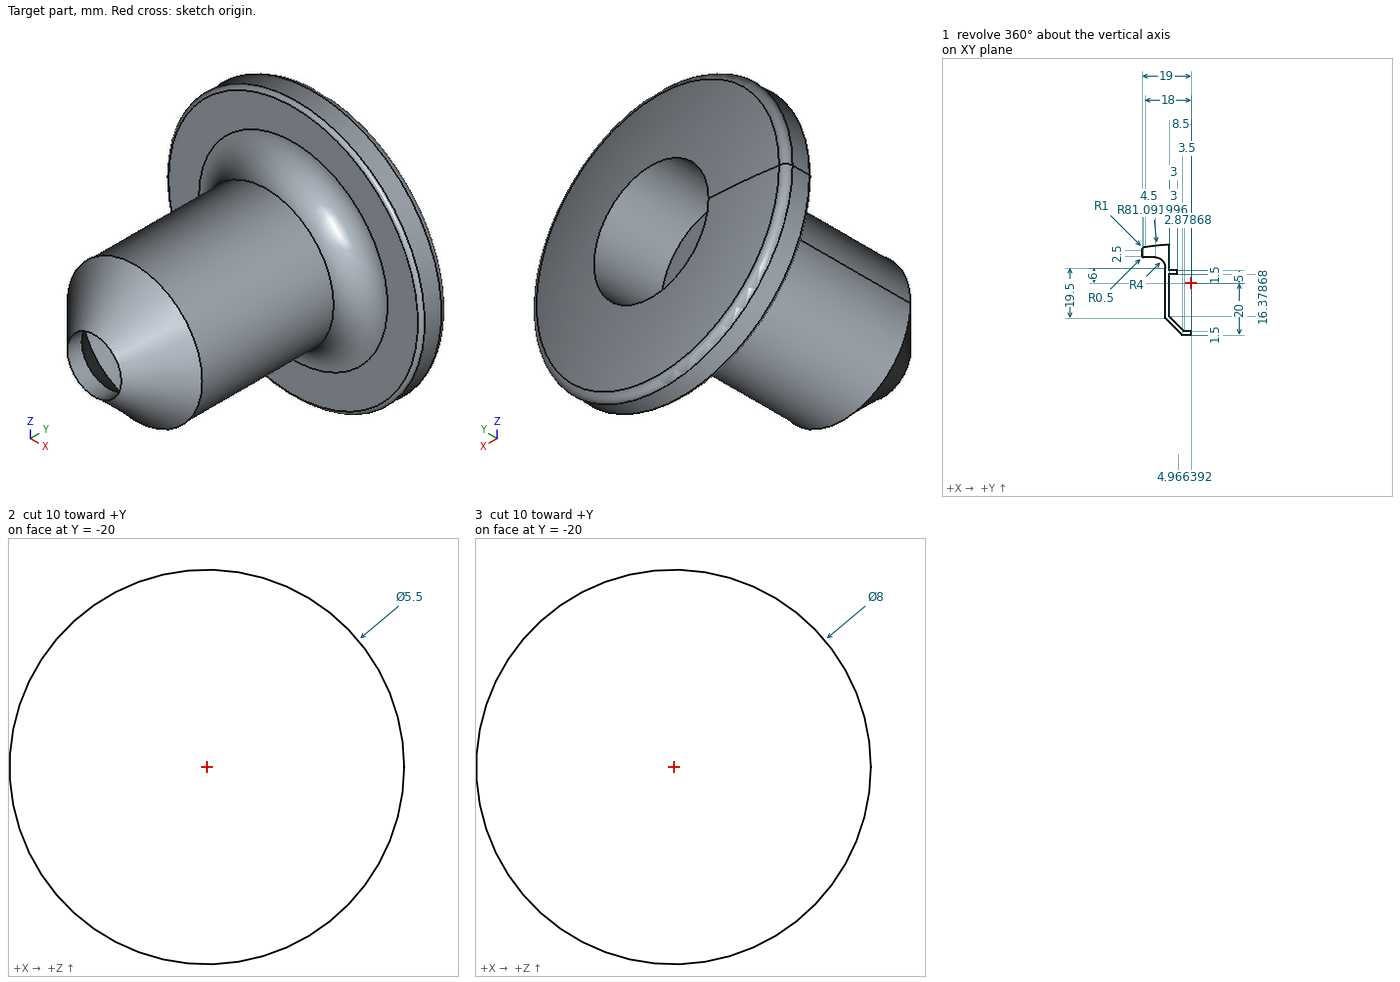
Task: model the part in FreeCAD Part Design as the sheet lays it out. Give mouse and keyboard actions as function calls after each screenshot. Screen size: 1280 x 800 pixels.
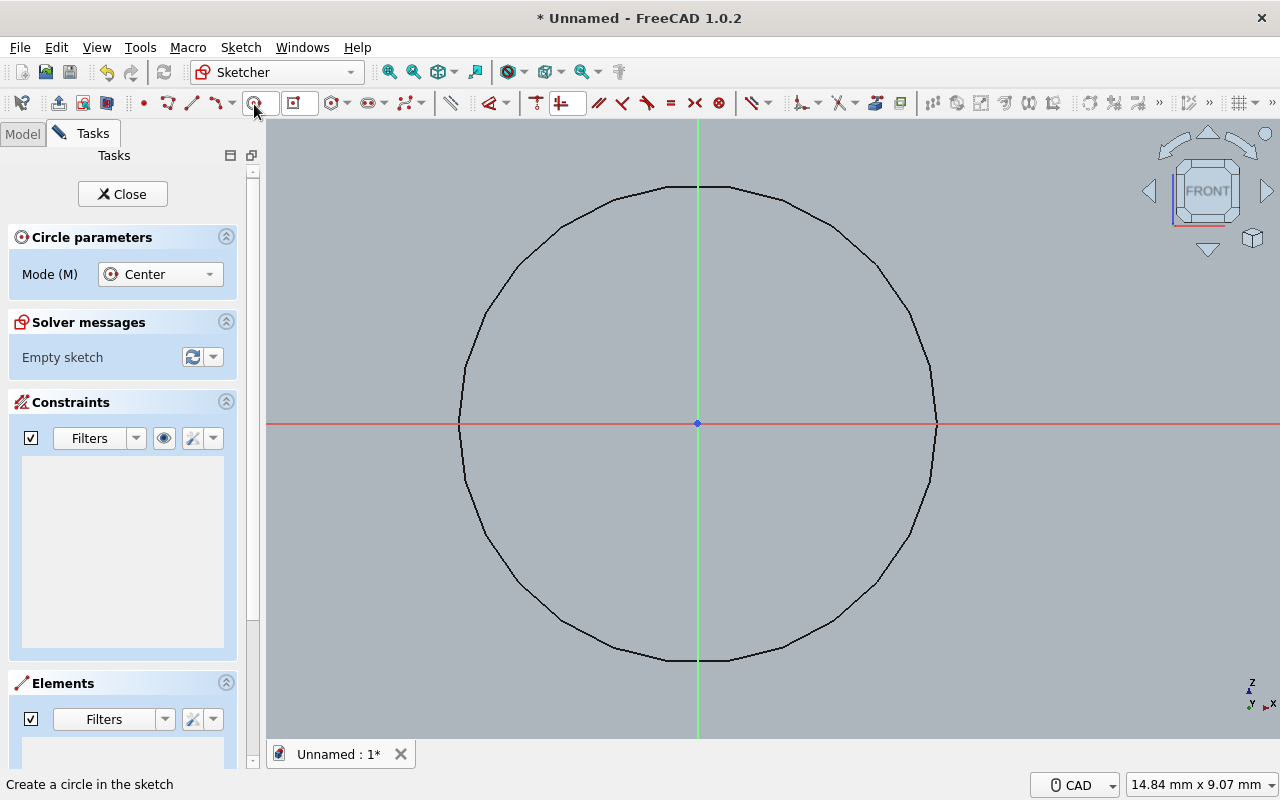
click(698, 424)
move(831, 291)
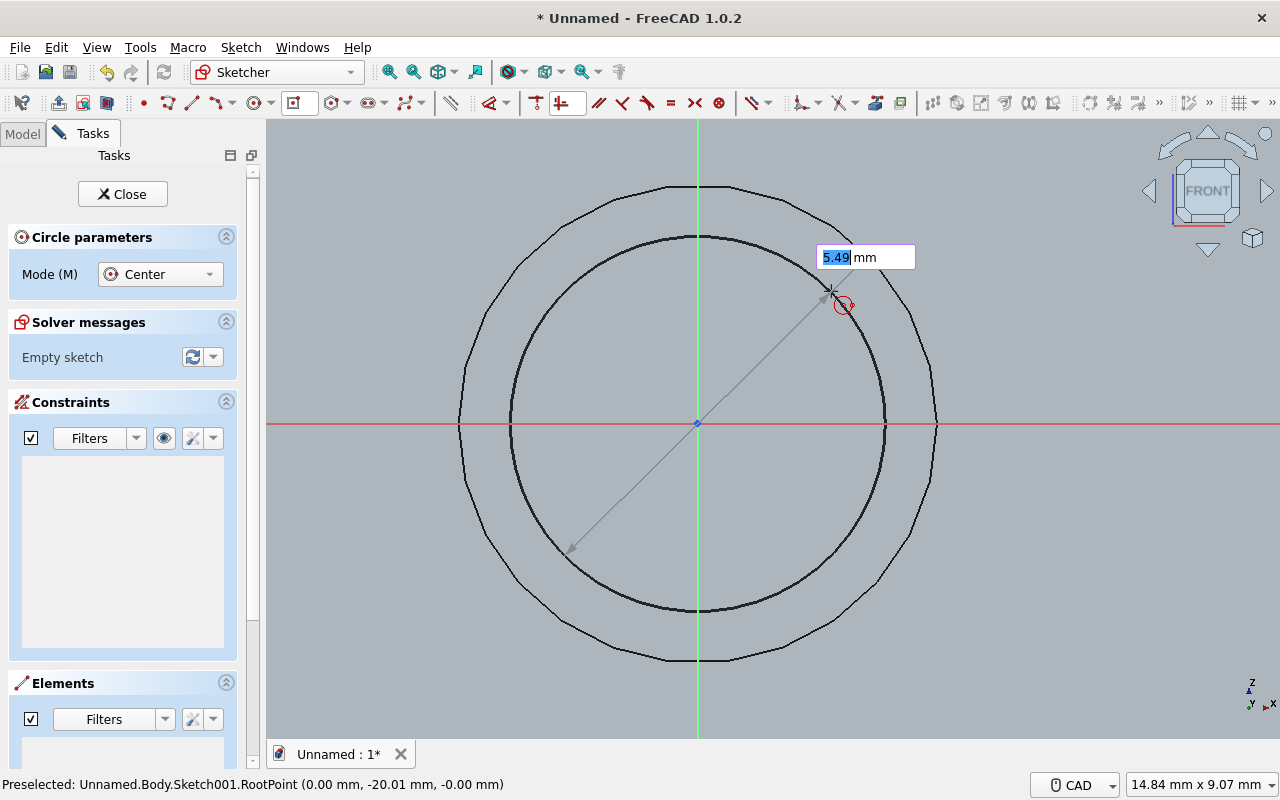
text(5.5)
key(Return)
key(Escape)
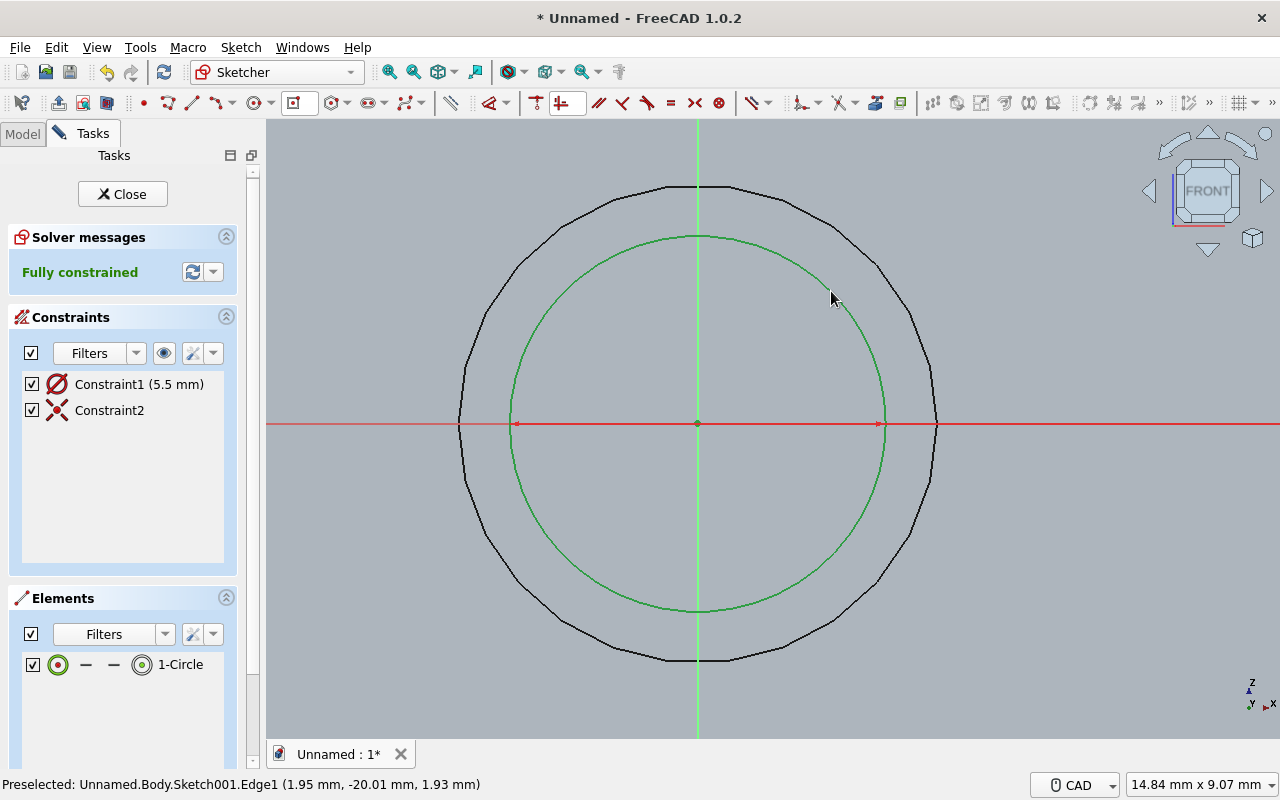
click(123, 194)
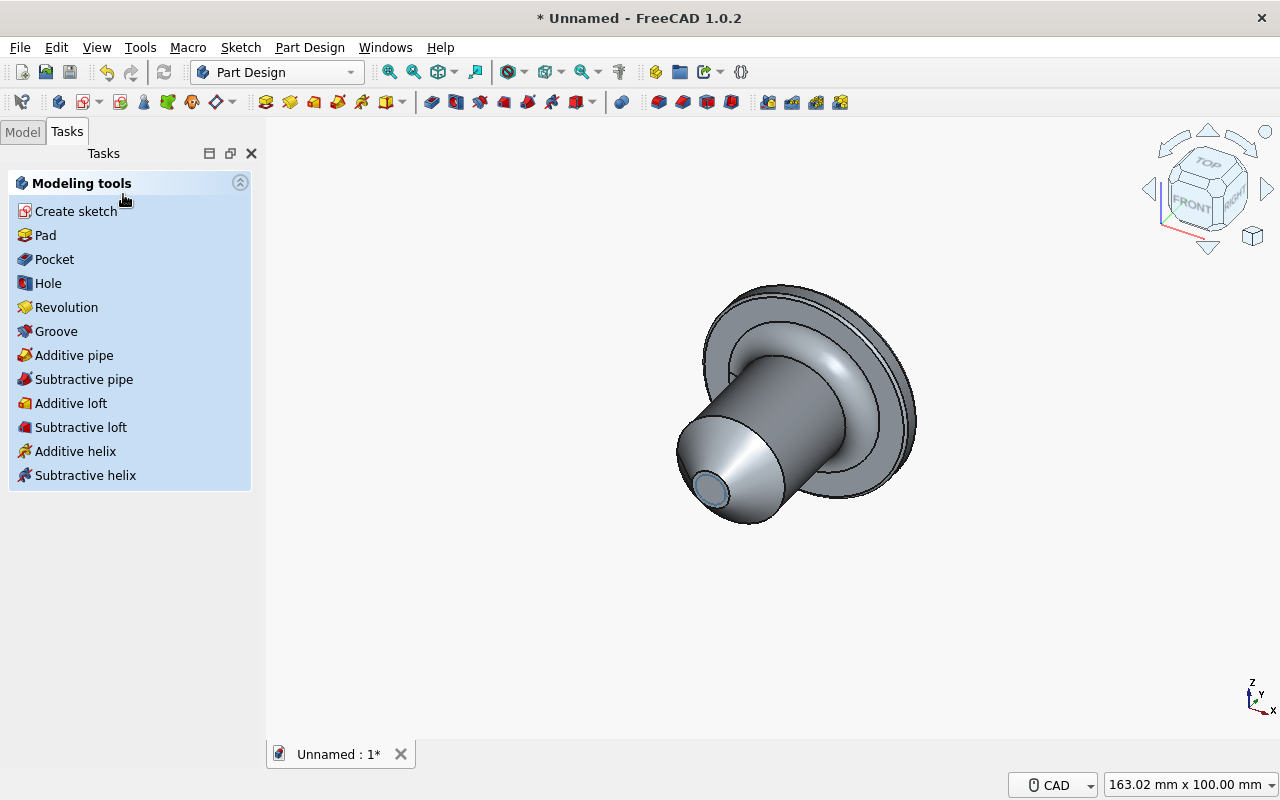
click(432, 102)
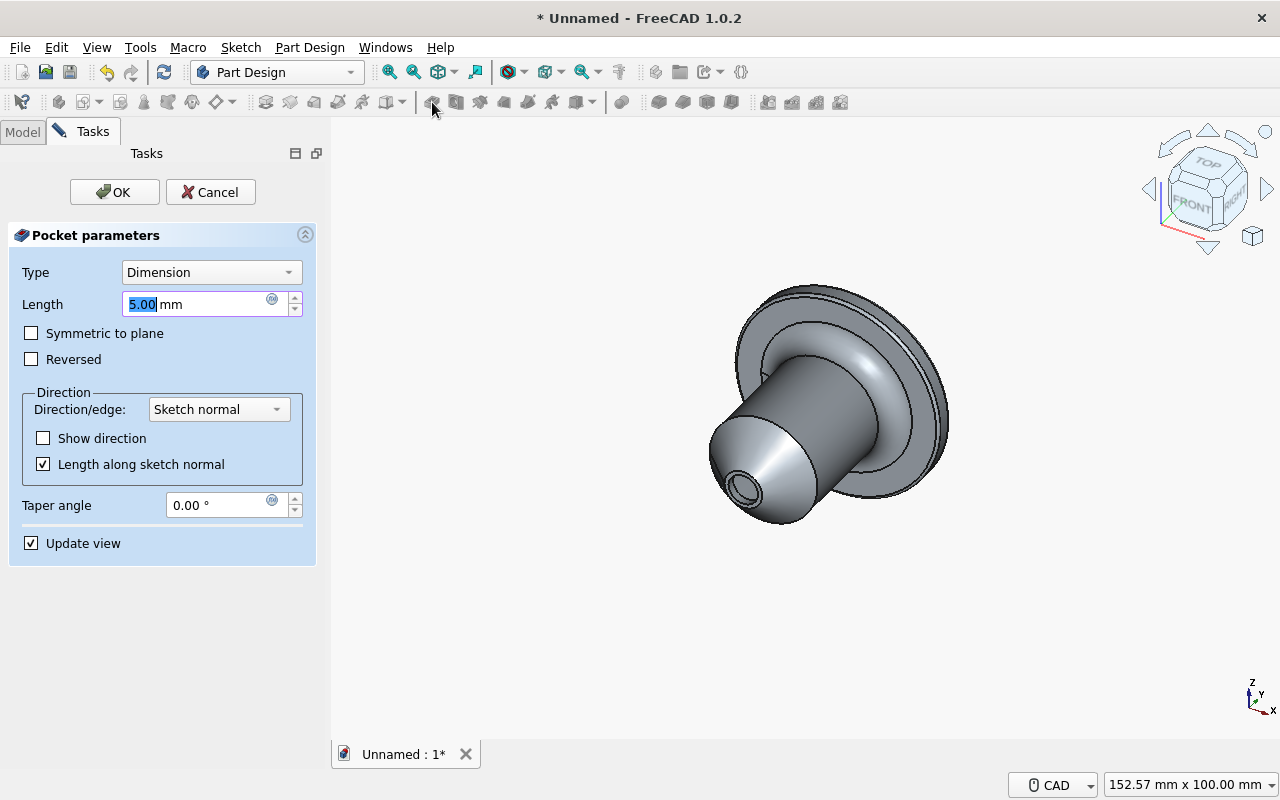
text(10)
key(Tab)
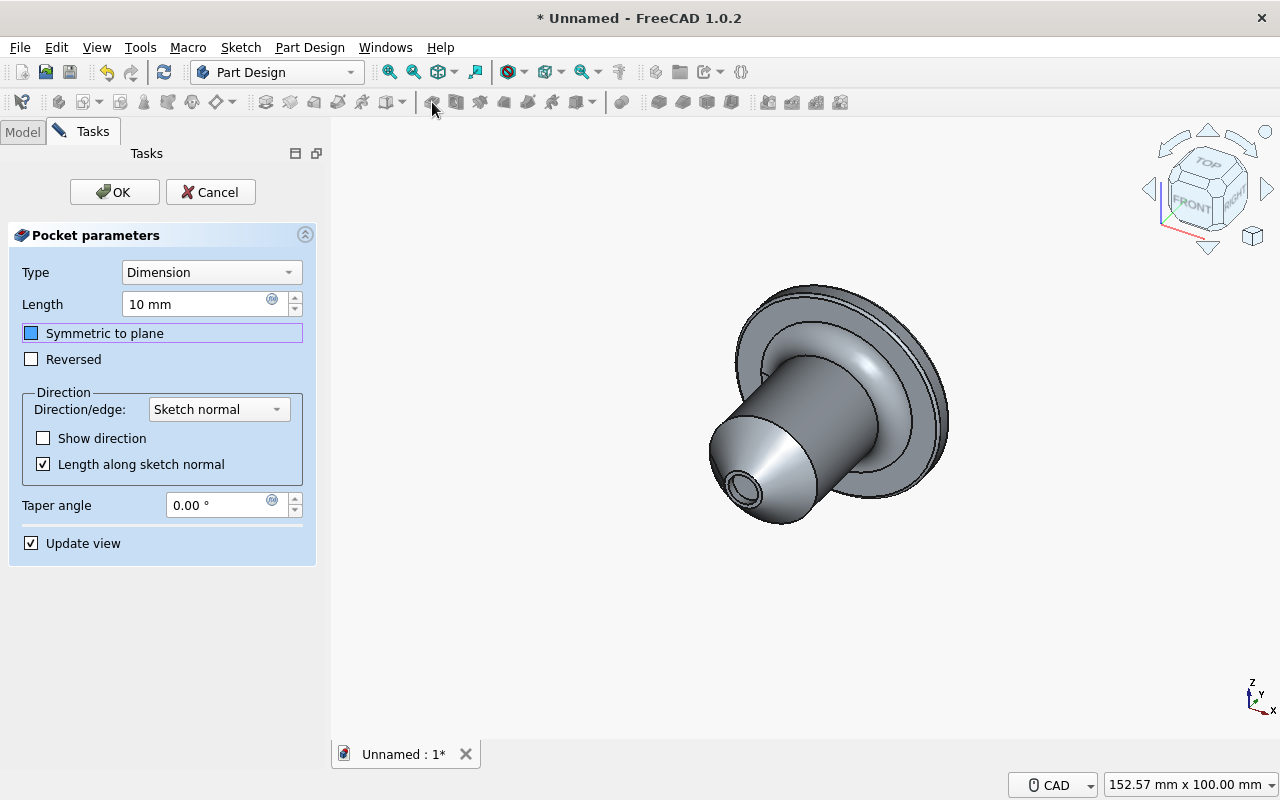
click(115, 192)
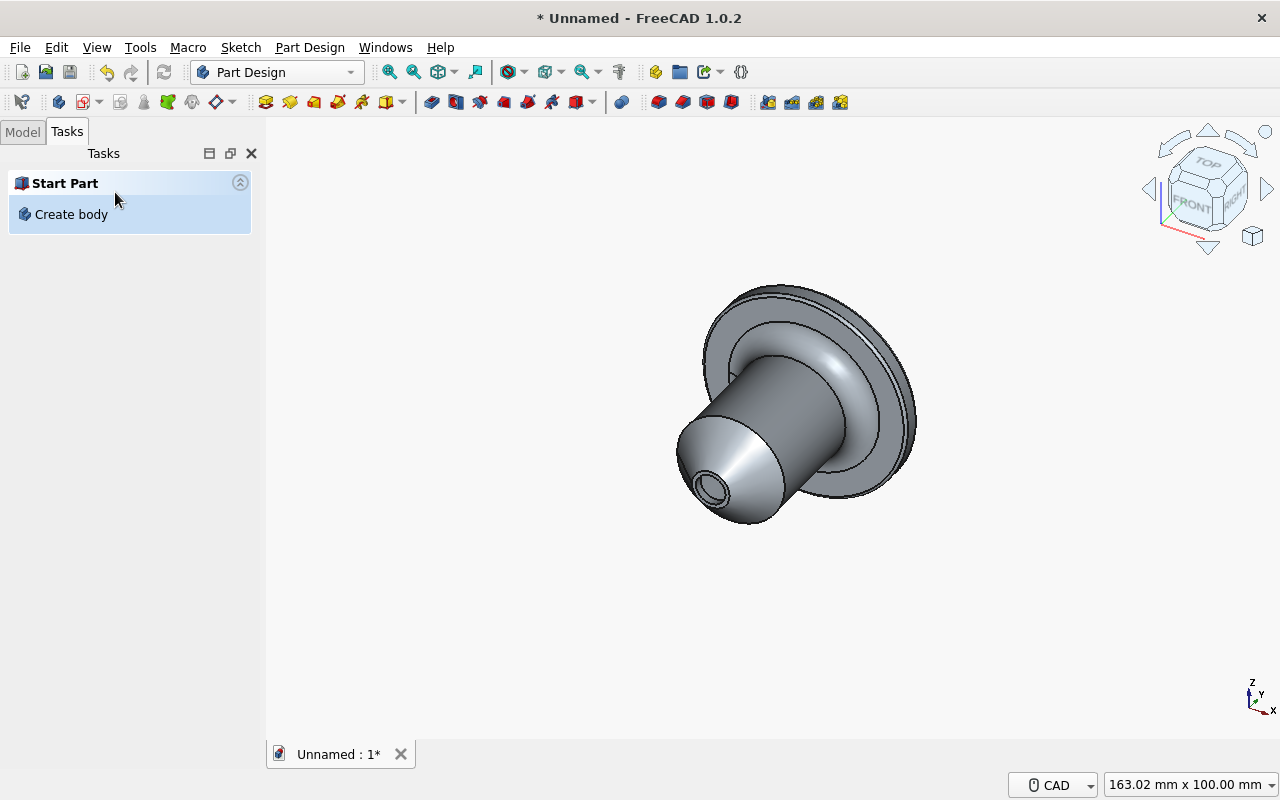
scroll(727, 499, up, 9)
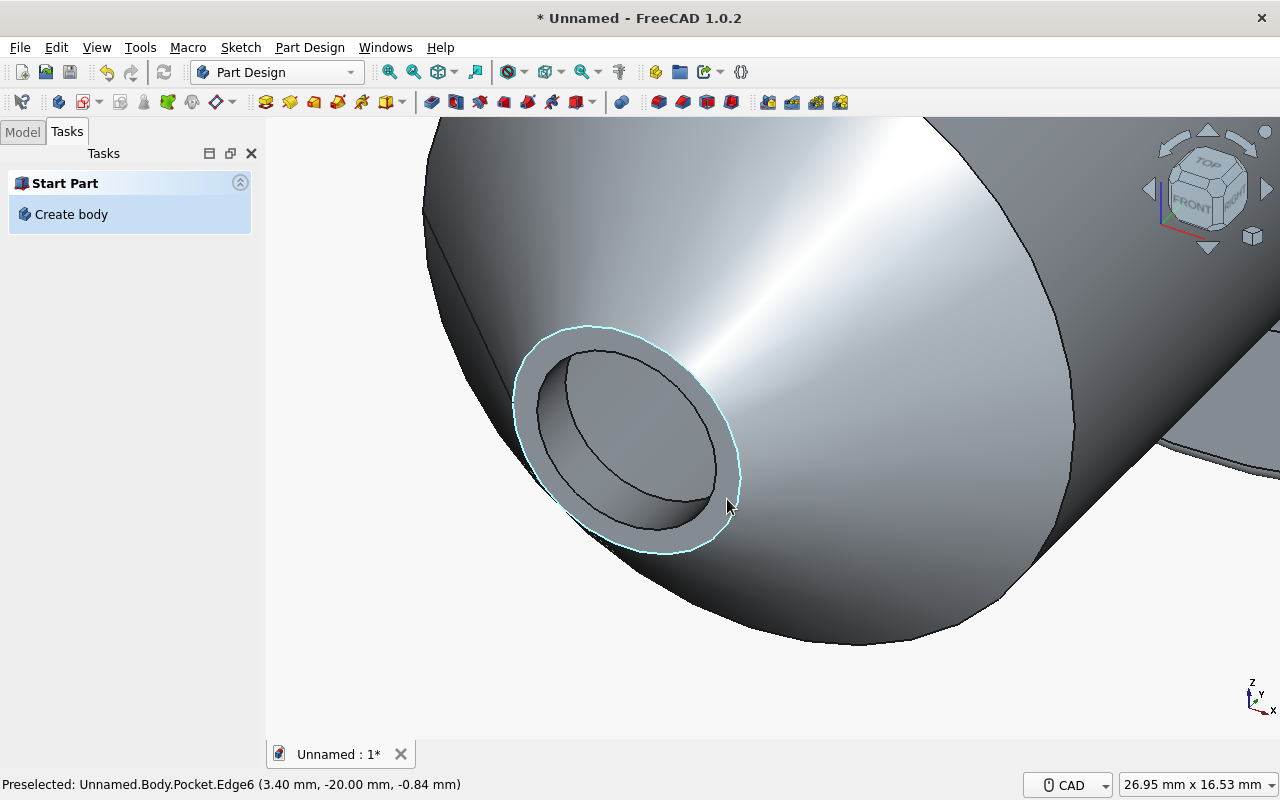
click(724, 502)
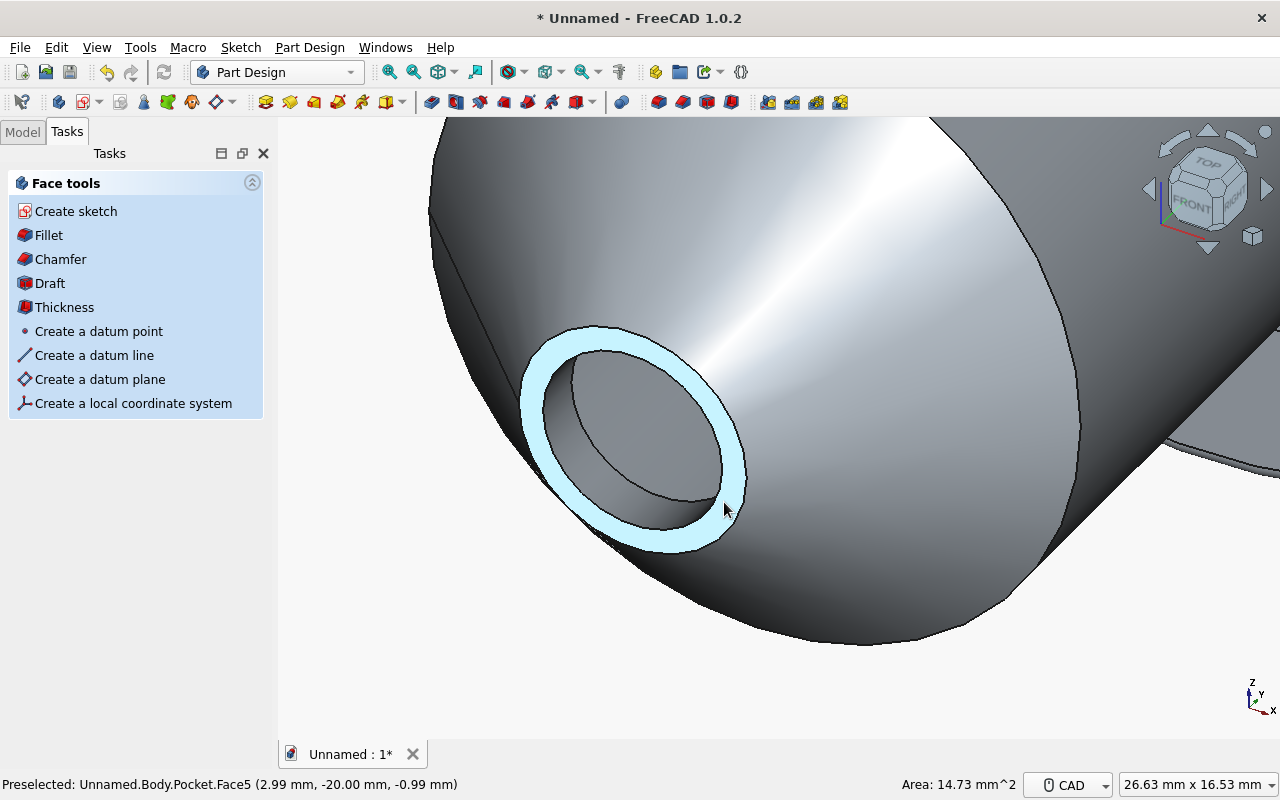
click(84, 102)